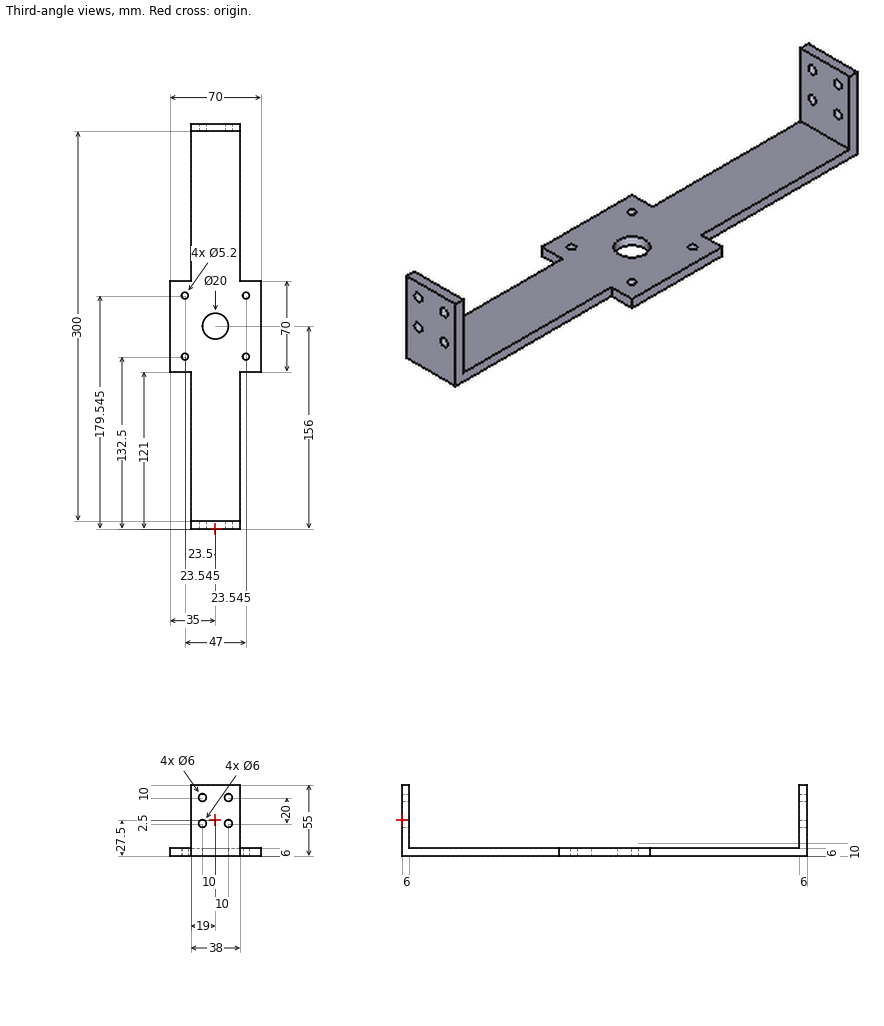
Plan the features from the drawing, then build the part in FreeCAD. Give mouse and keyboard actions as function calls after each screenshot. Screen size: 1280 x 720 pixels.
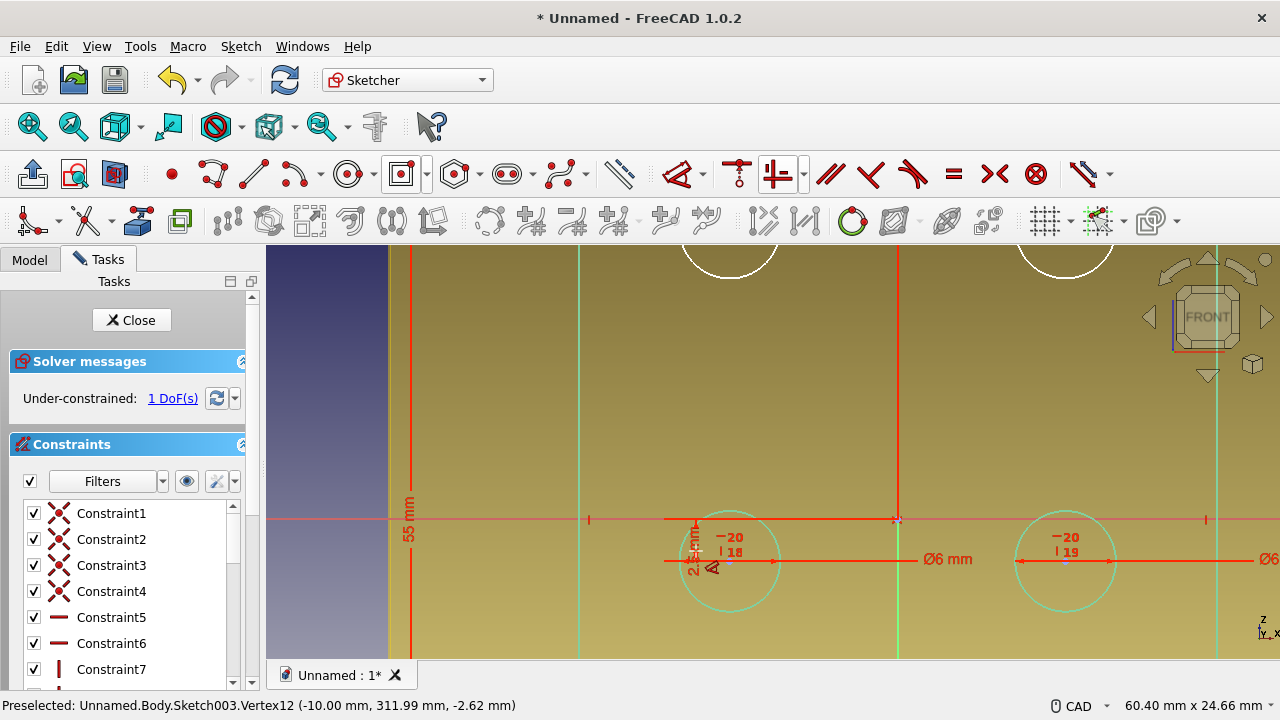
scroll(621, 423, down, 6)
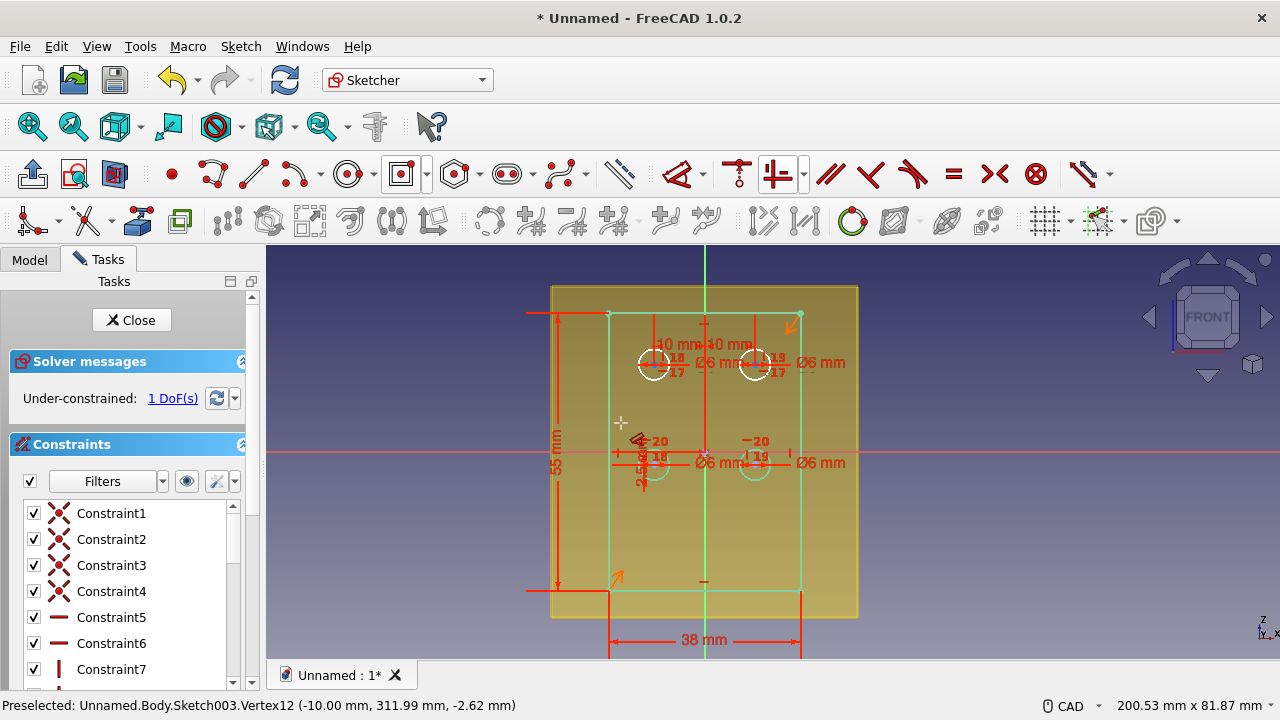
click(609, 313)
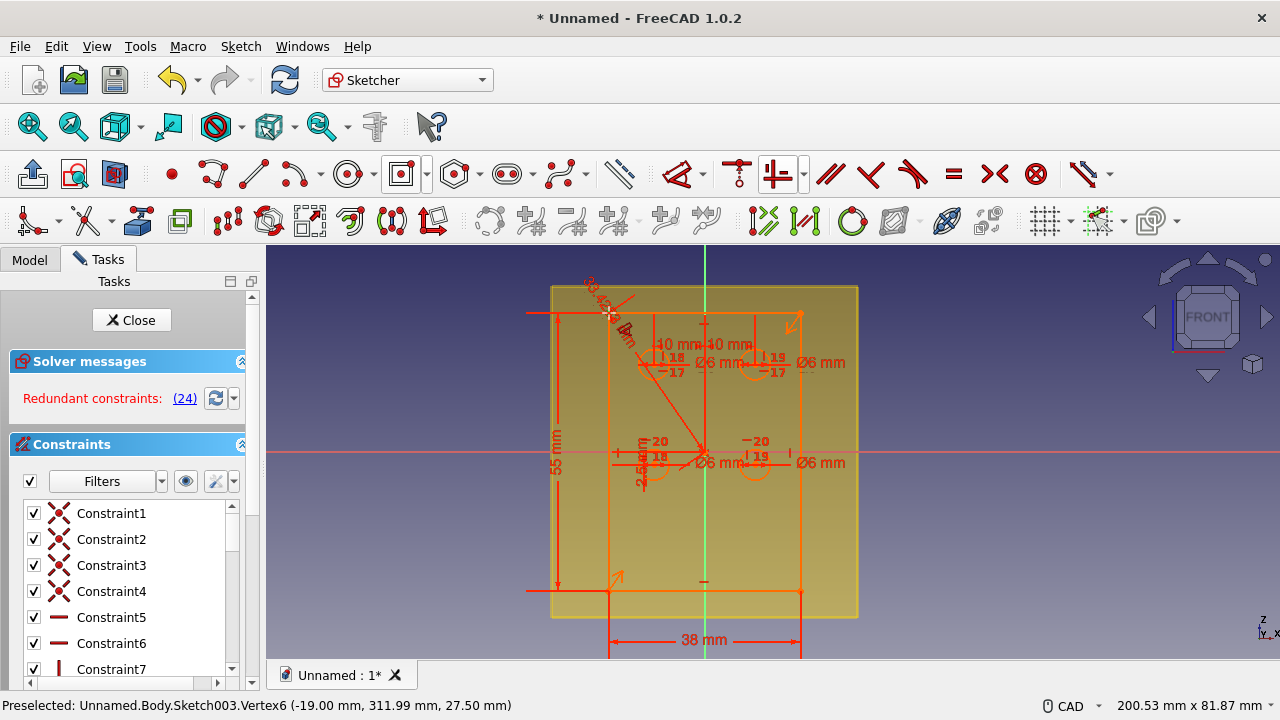
click(654, 365)
click(575, 339)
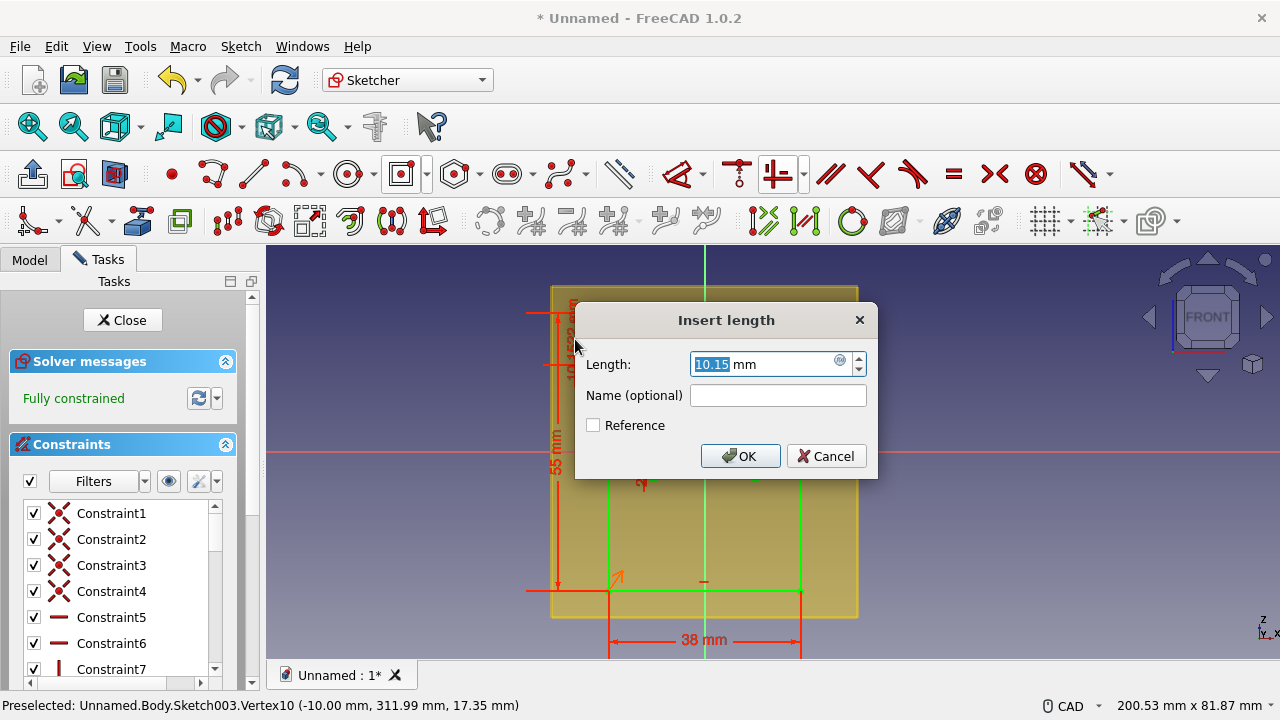
text(10)
key(Return)
key(Escape)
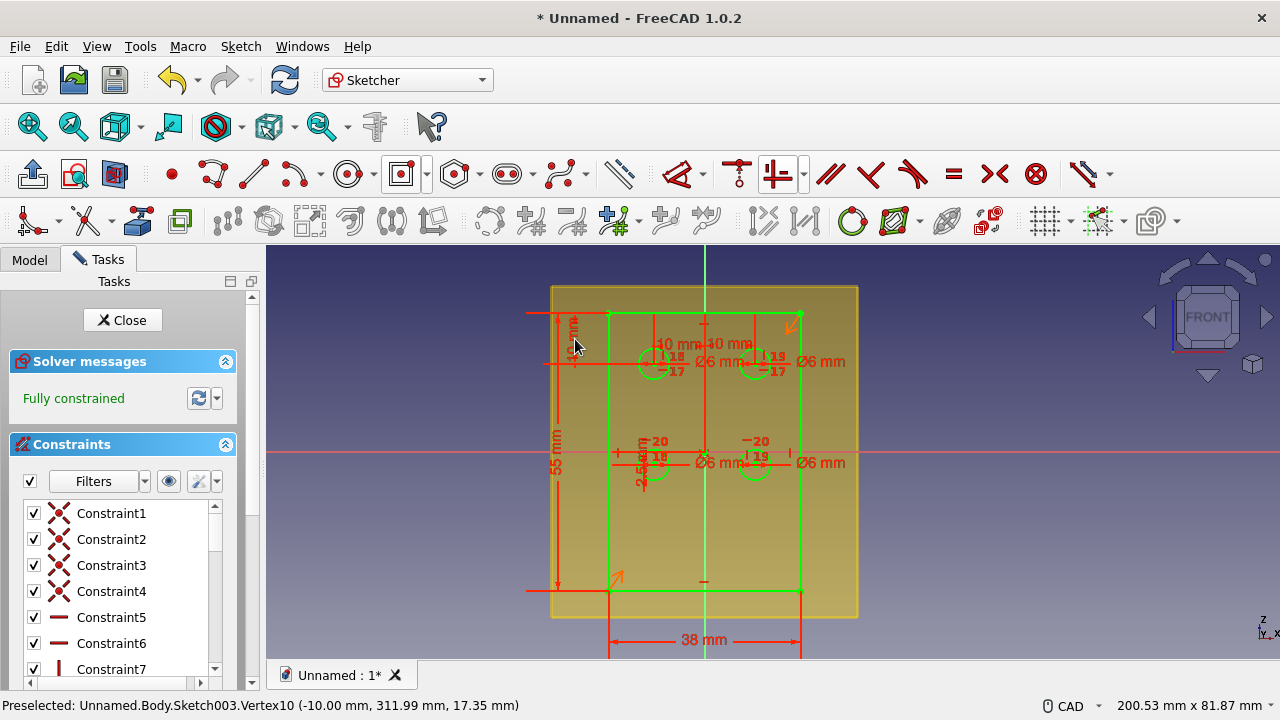
click(123, 320)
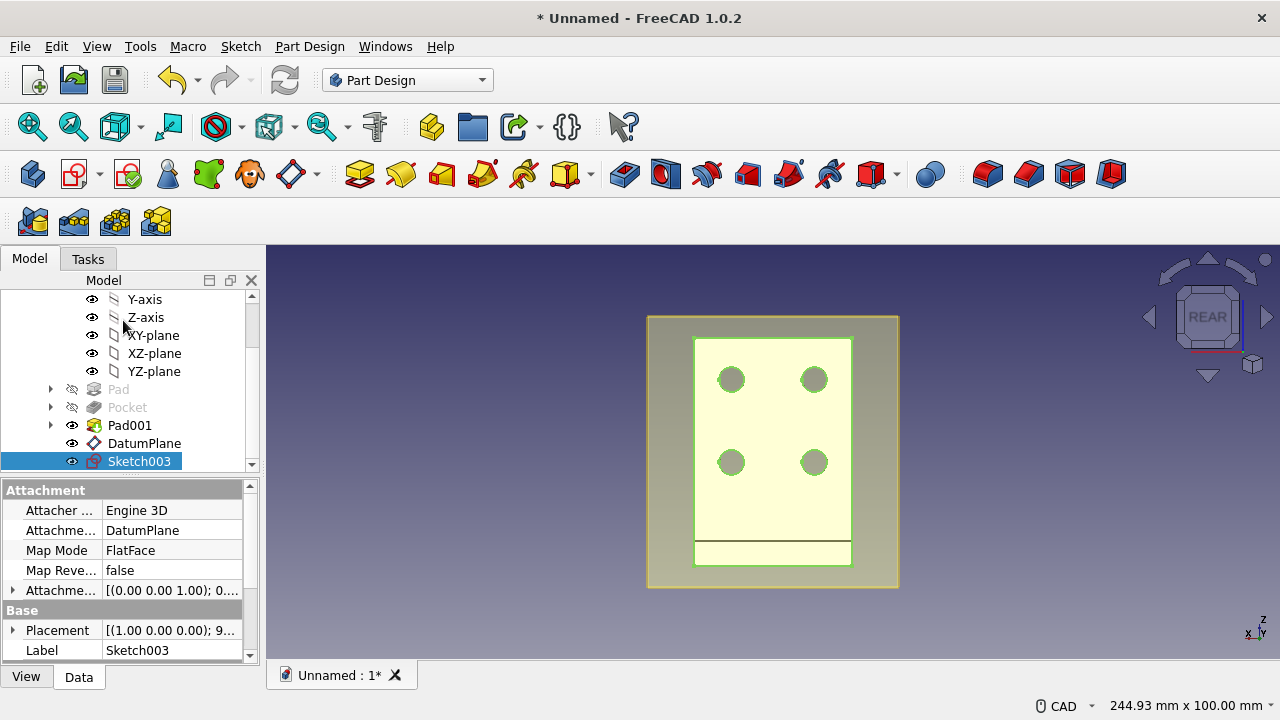
click(360, 174)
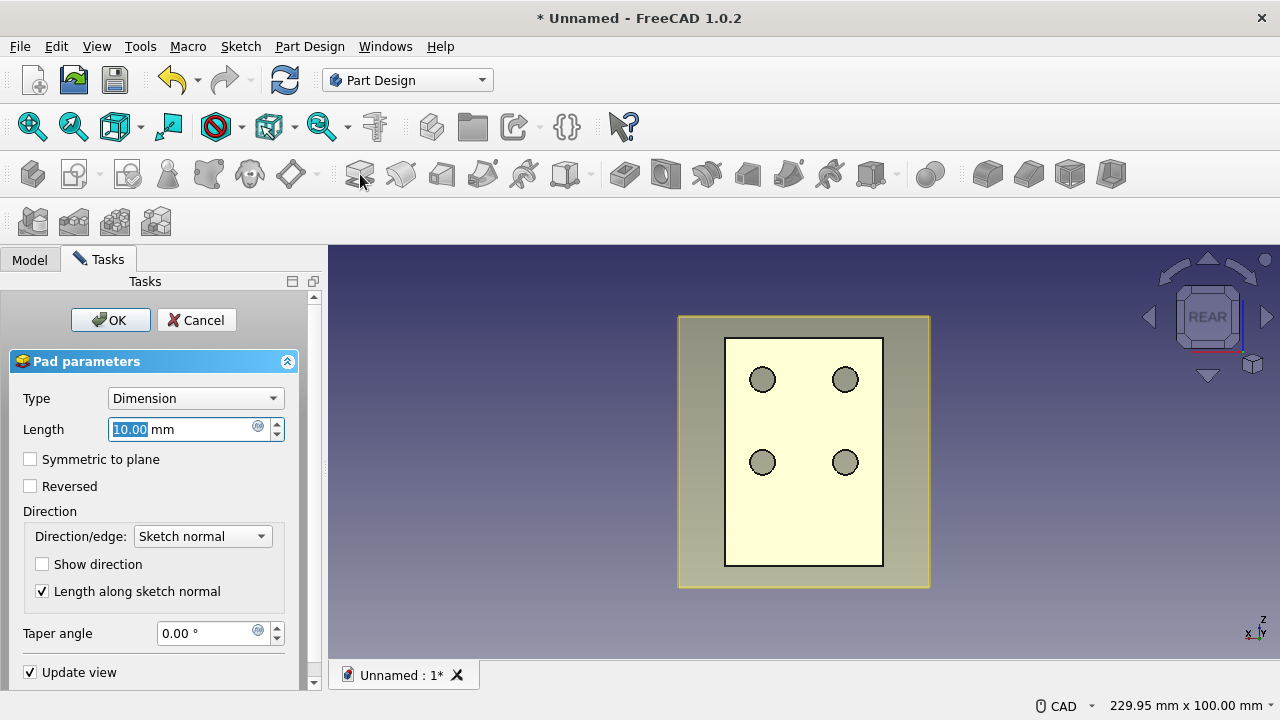
text(6)
key(Tab)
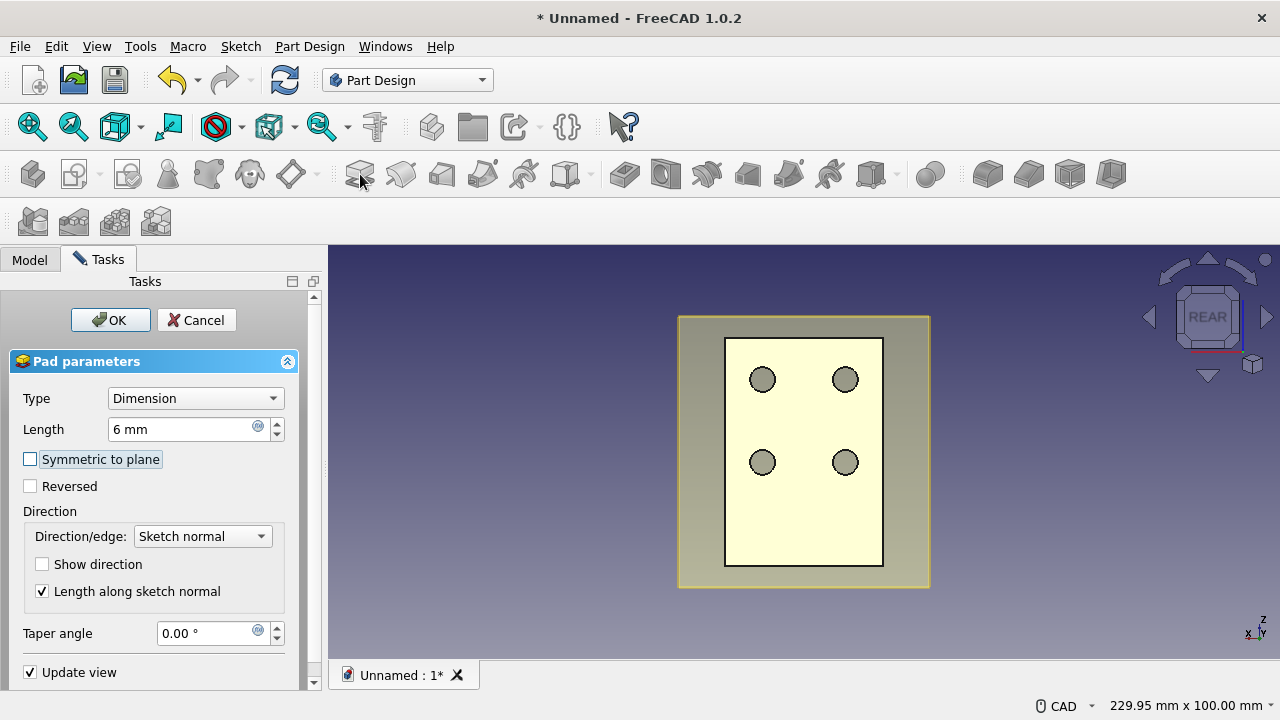
click(111, 320)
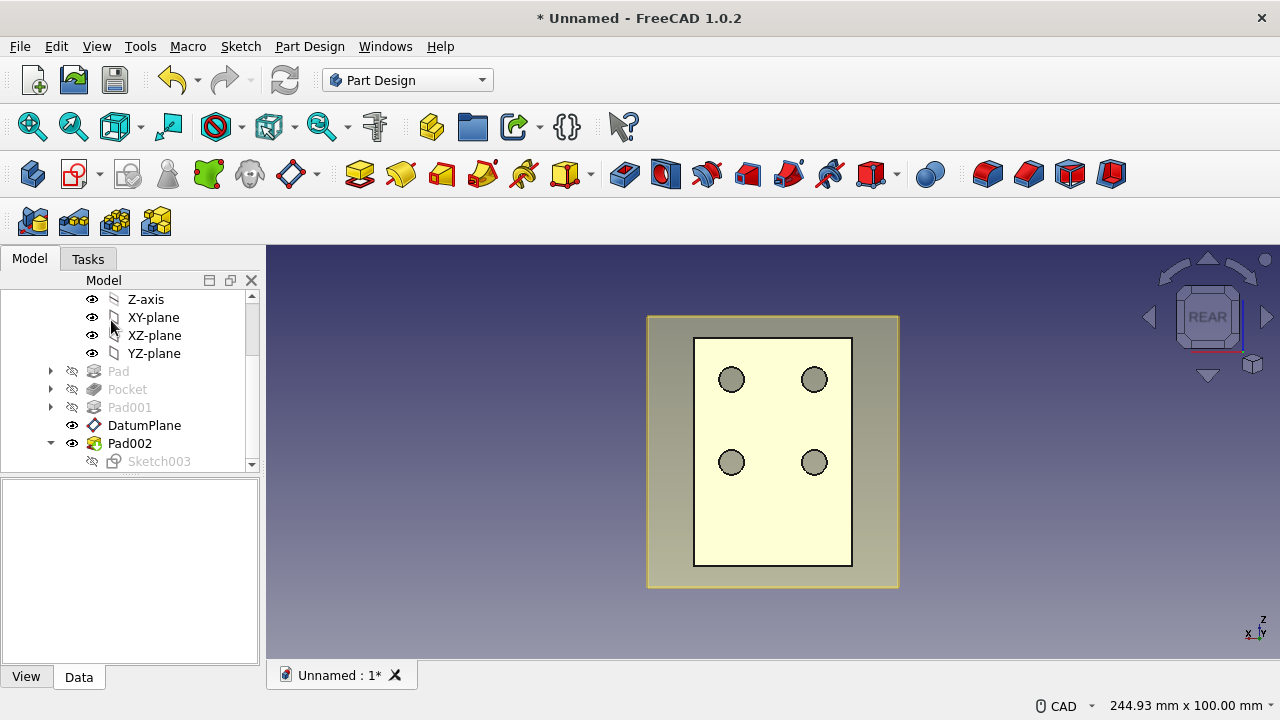
click(117, 425)
key(space)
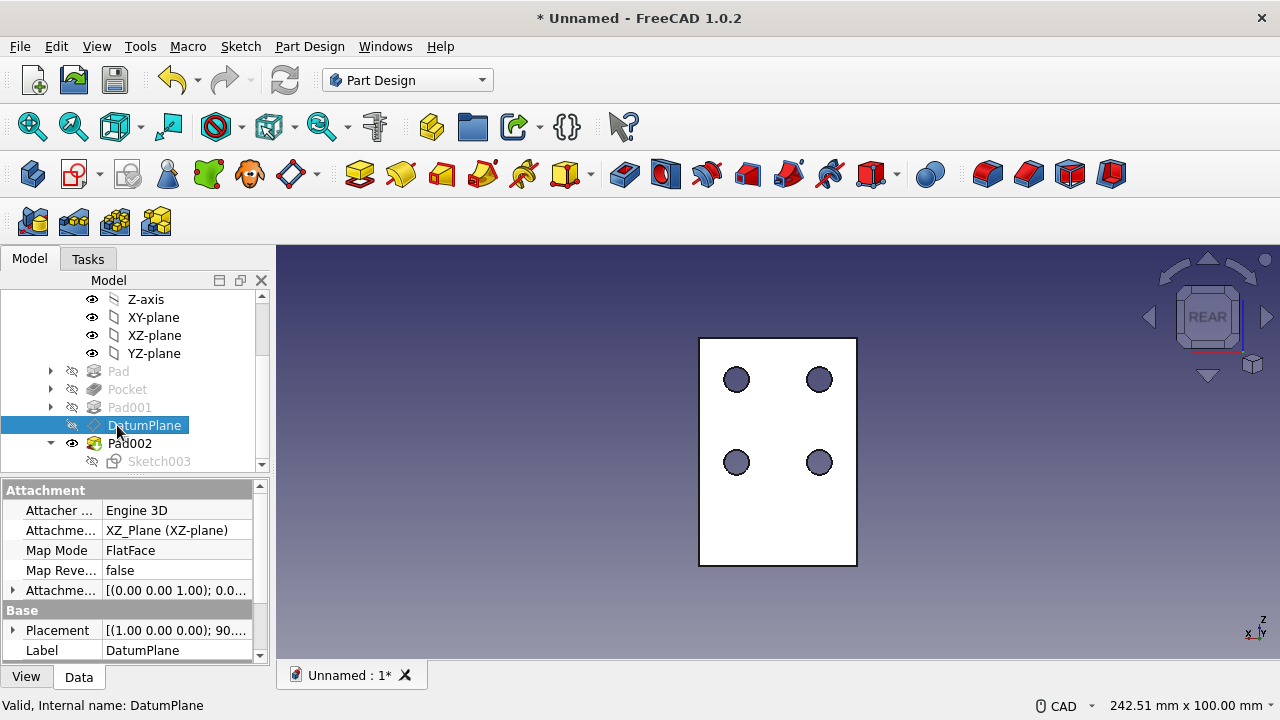
key(5)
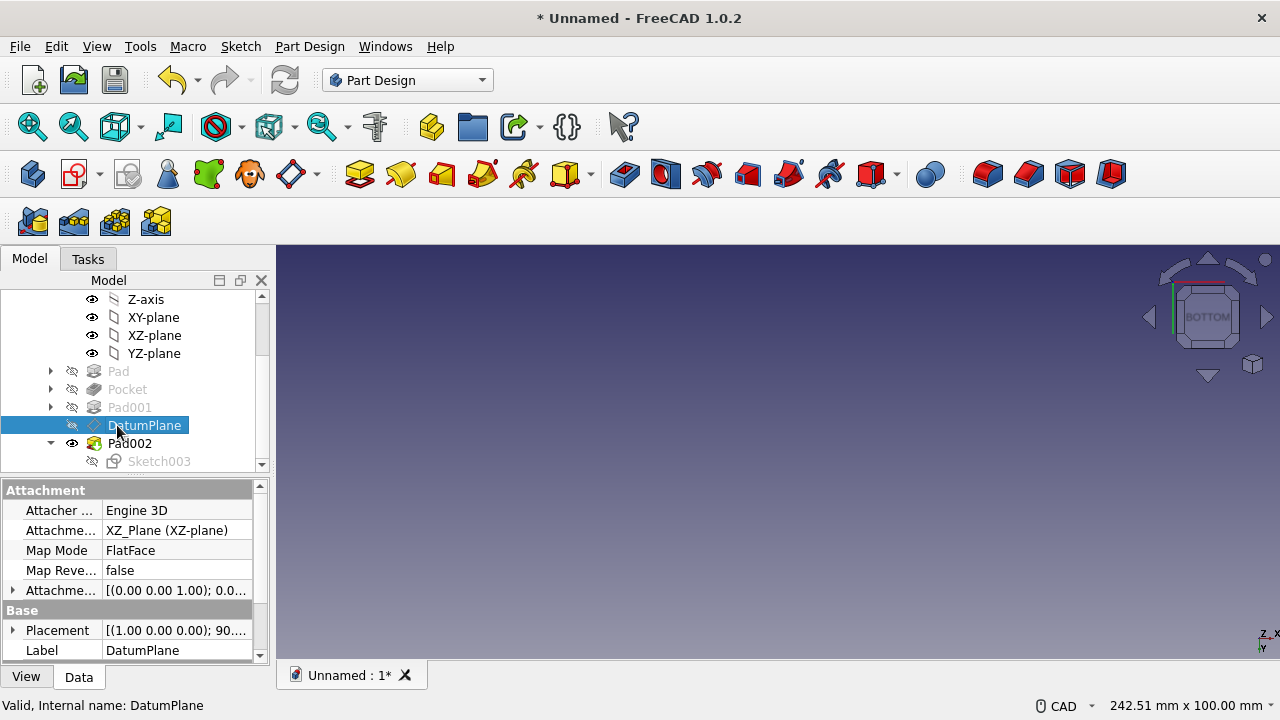
key(v)
key(f)